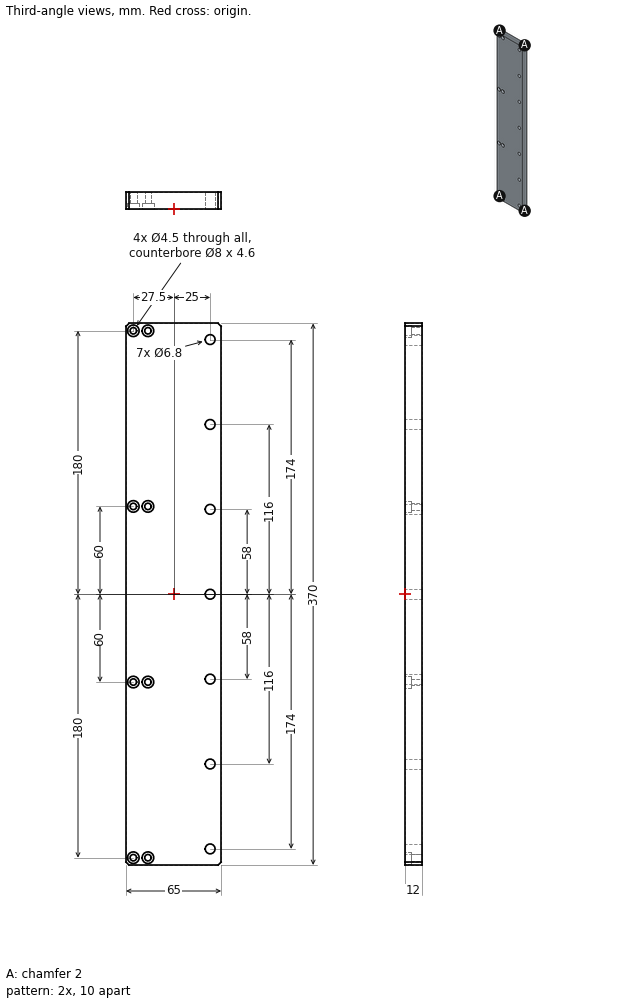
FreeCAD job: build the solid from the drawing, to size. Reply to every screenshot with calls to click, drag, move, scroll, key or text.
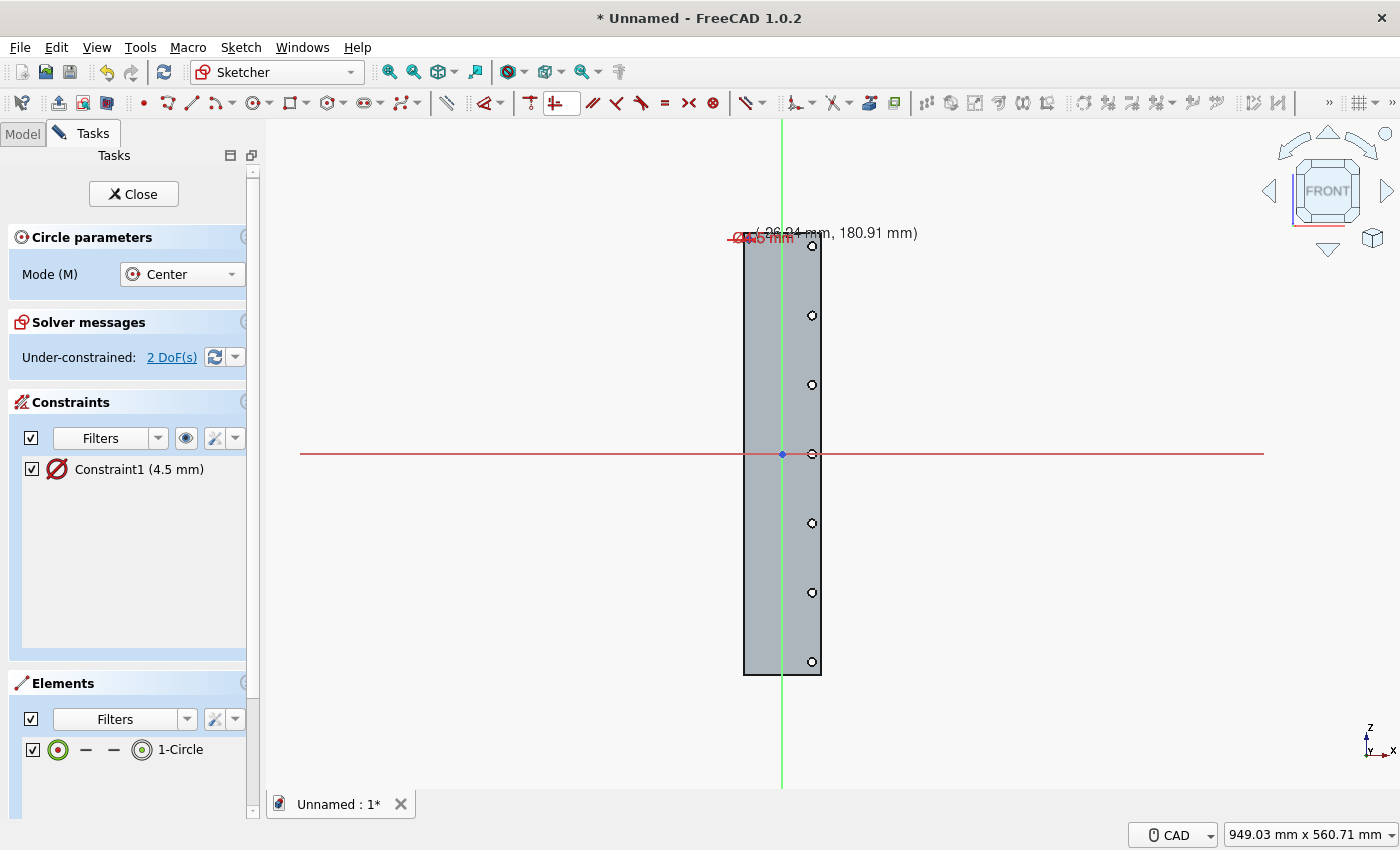
scroll(749, 382, up, 11)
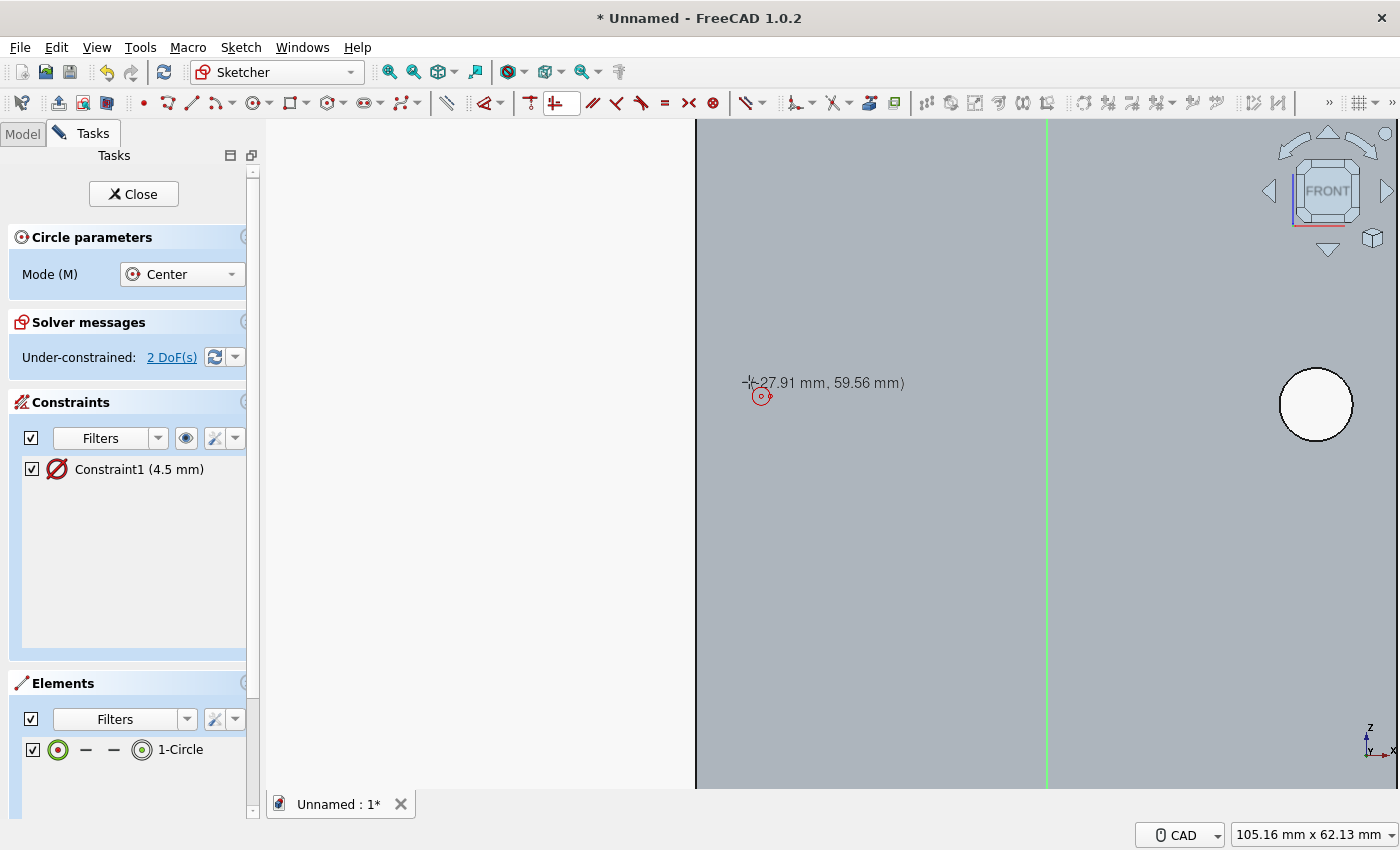
scroll(749, 382, down, 11)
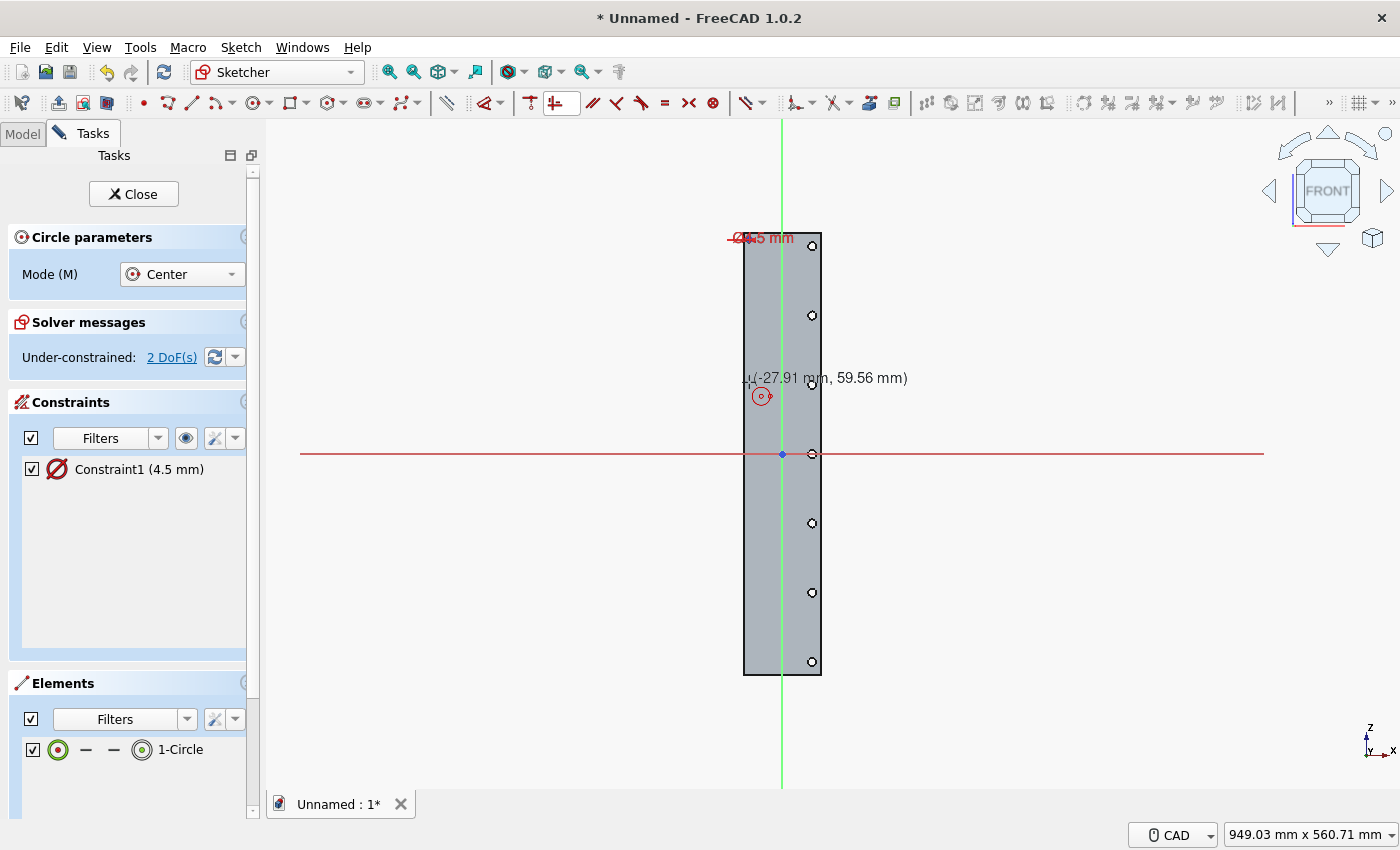
click(749, 382)
move(751, 381)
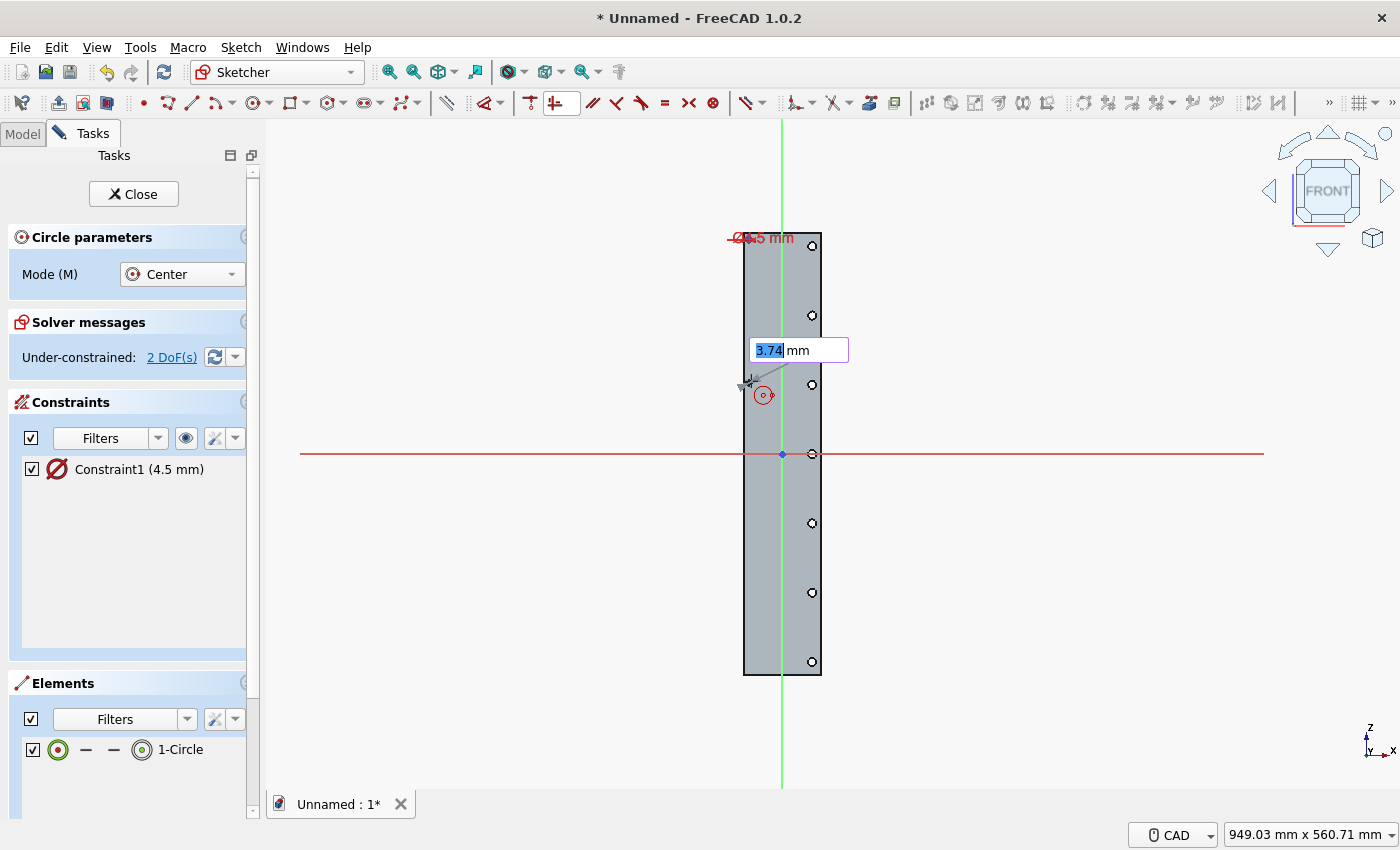
text(4.5)
key(Return)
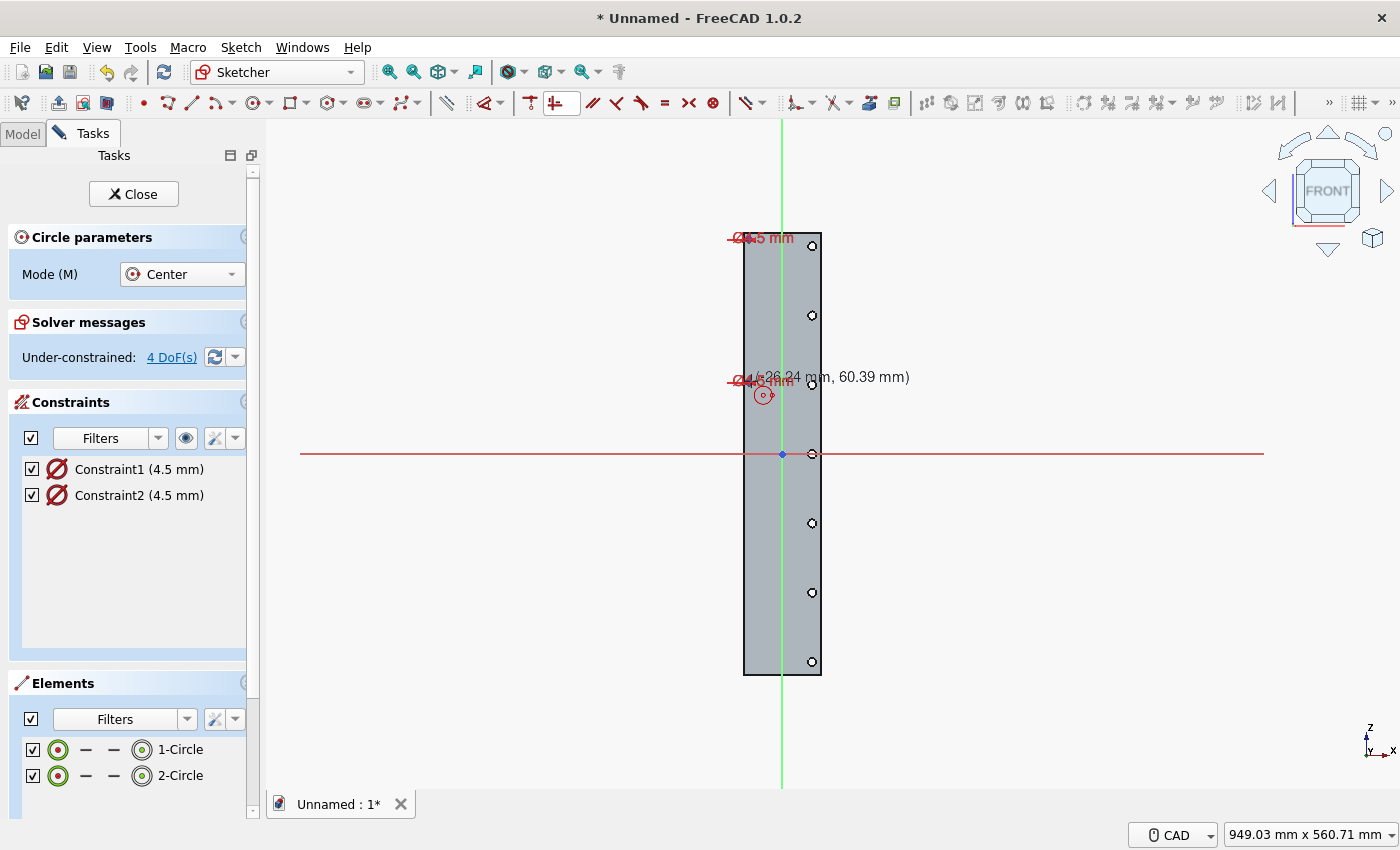
scroll(749, 526, up, 11)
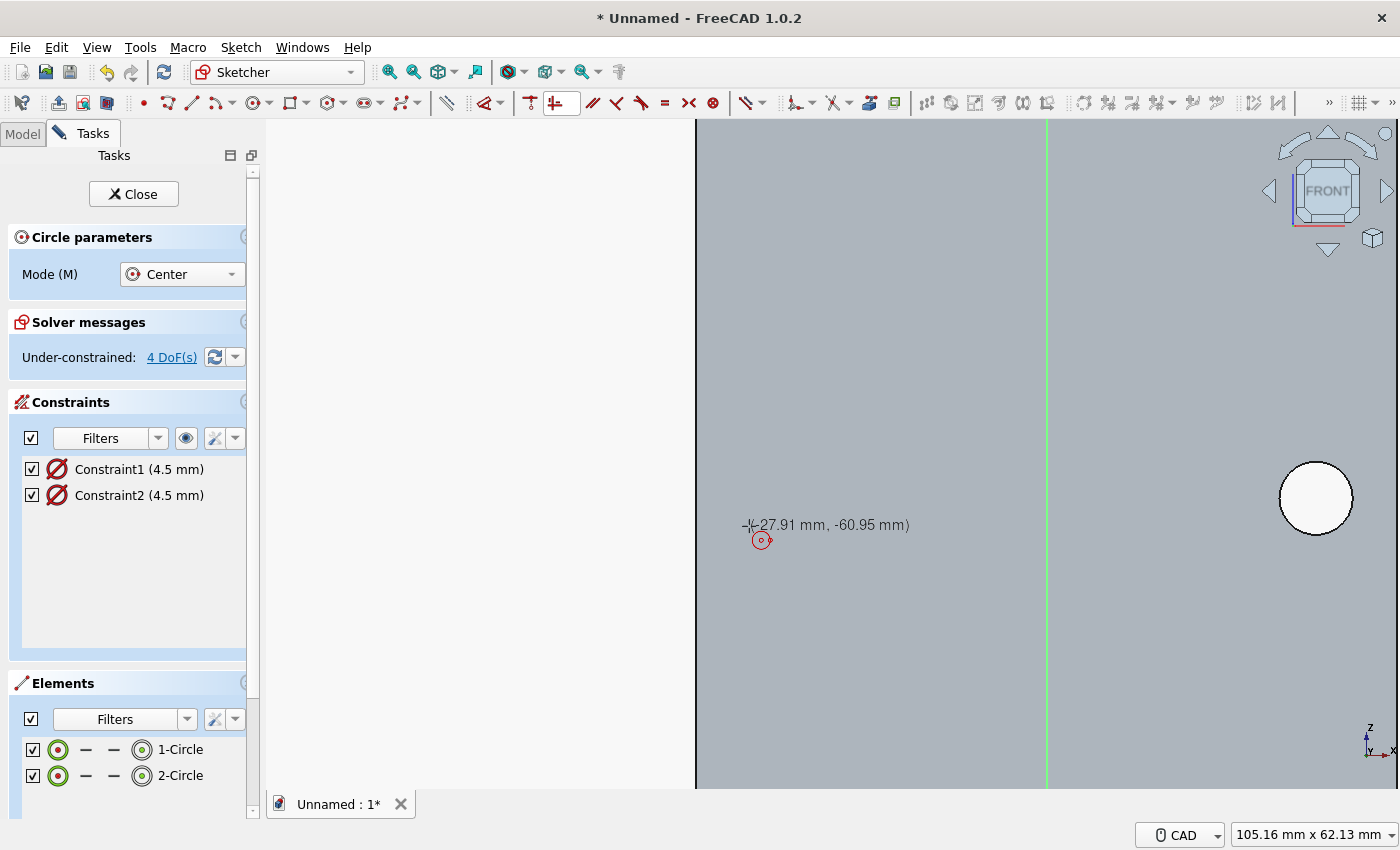
scroll(749, 526, down, 11)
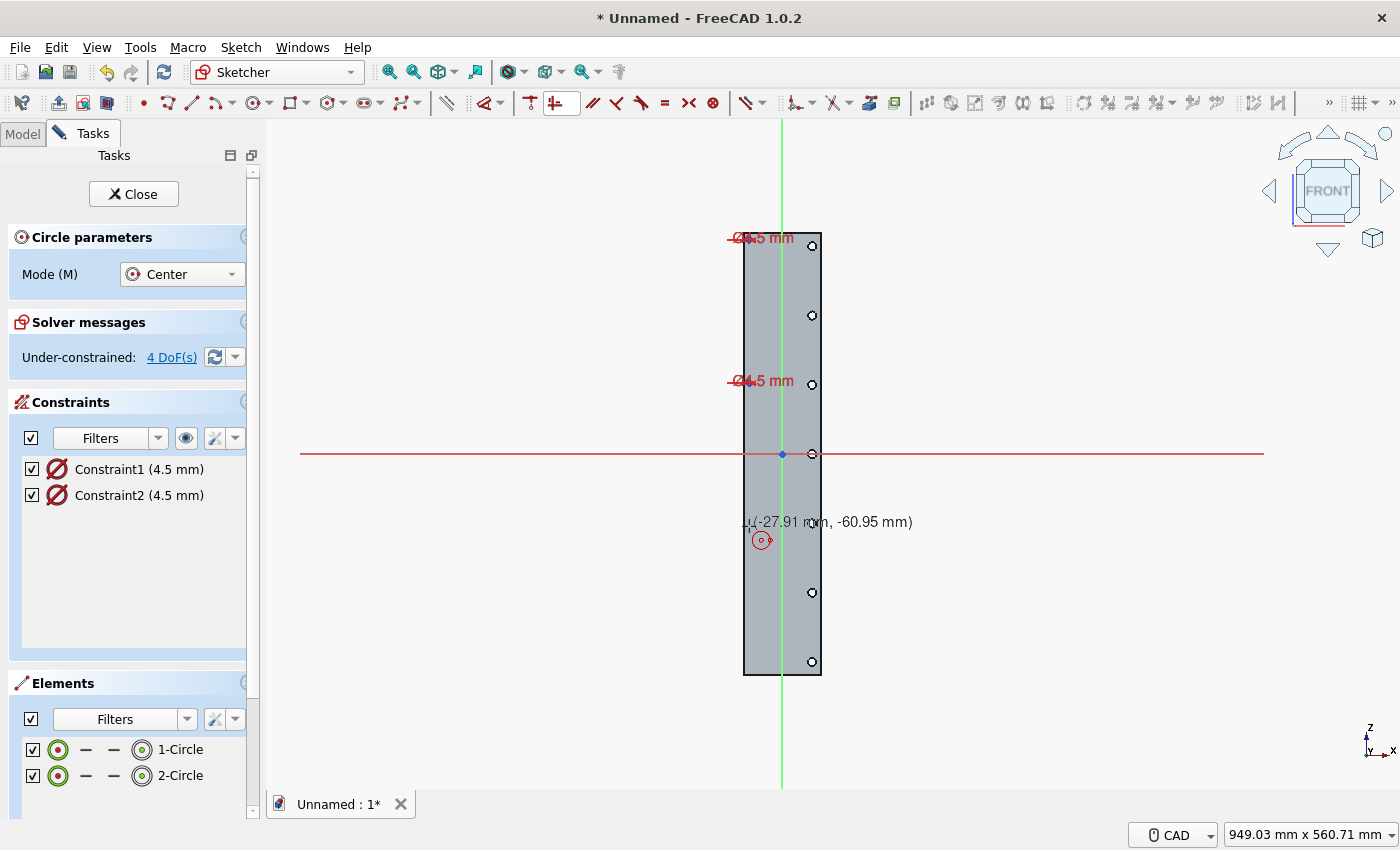
click(749, 526)
move(751, 524)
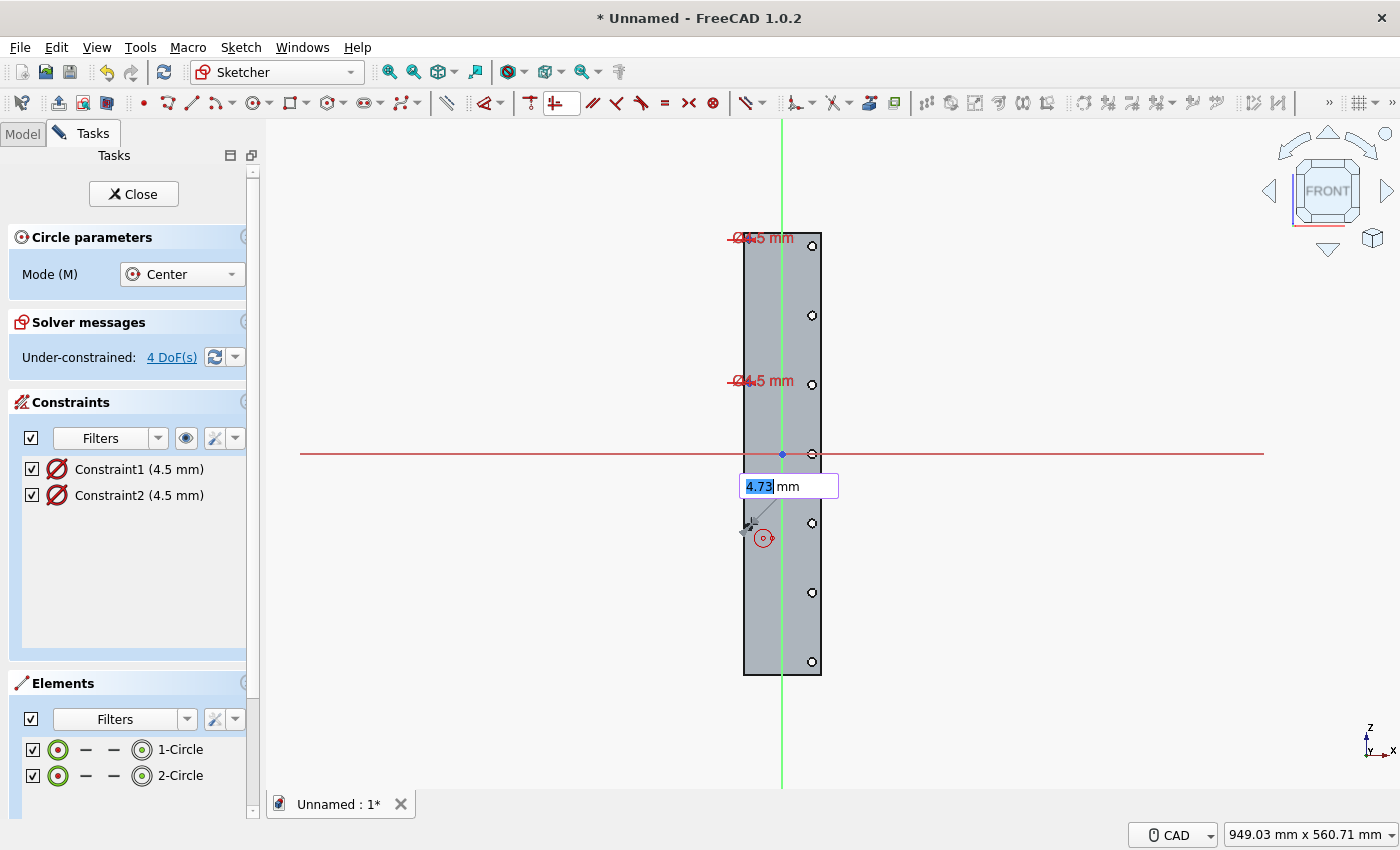
text(4.5)
key(Return)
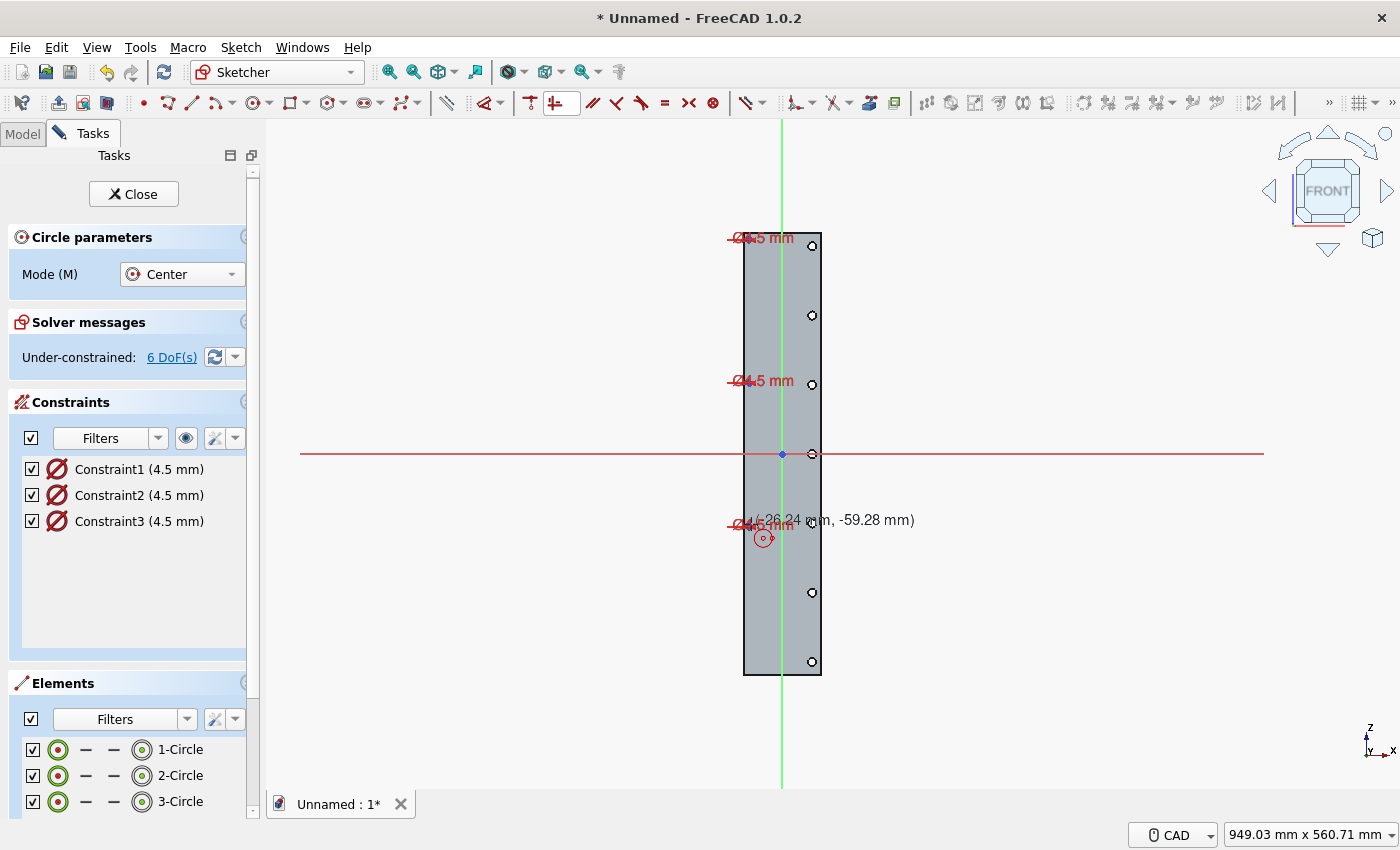
scroll(749, 669, up, 11)